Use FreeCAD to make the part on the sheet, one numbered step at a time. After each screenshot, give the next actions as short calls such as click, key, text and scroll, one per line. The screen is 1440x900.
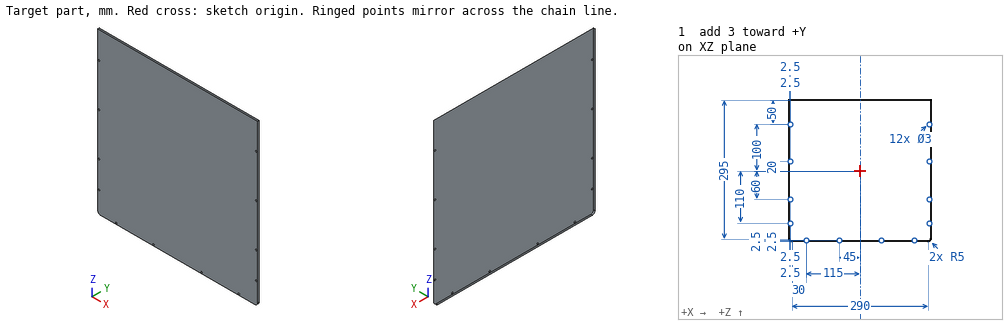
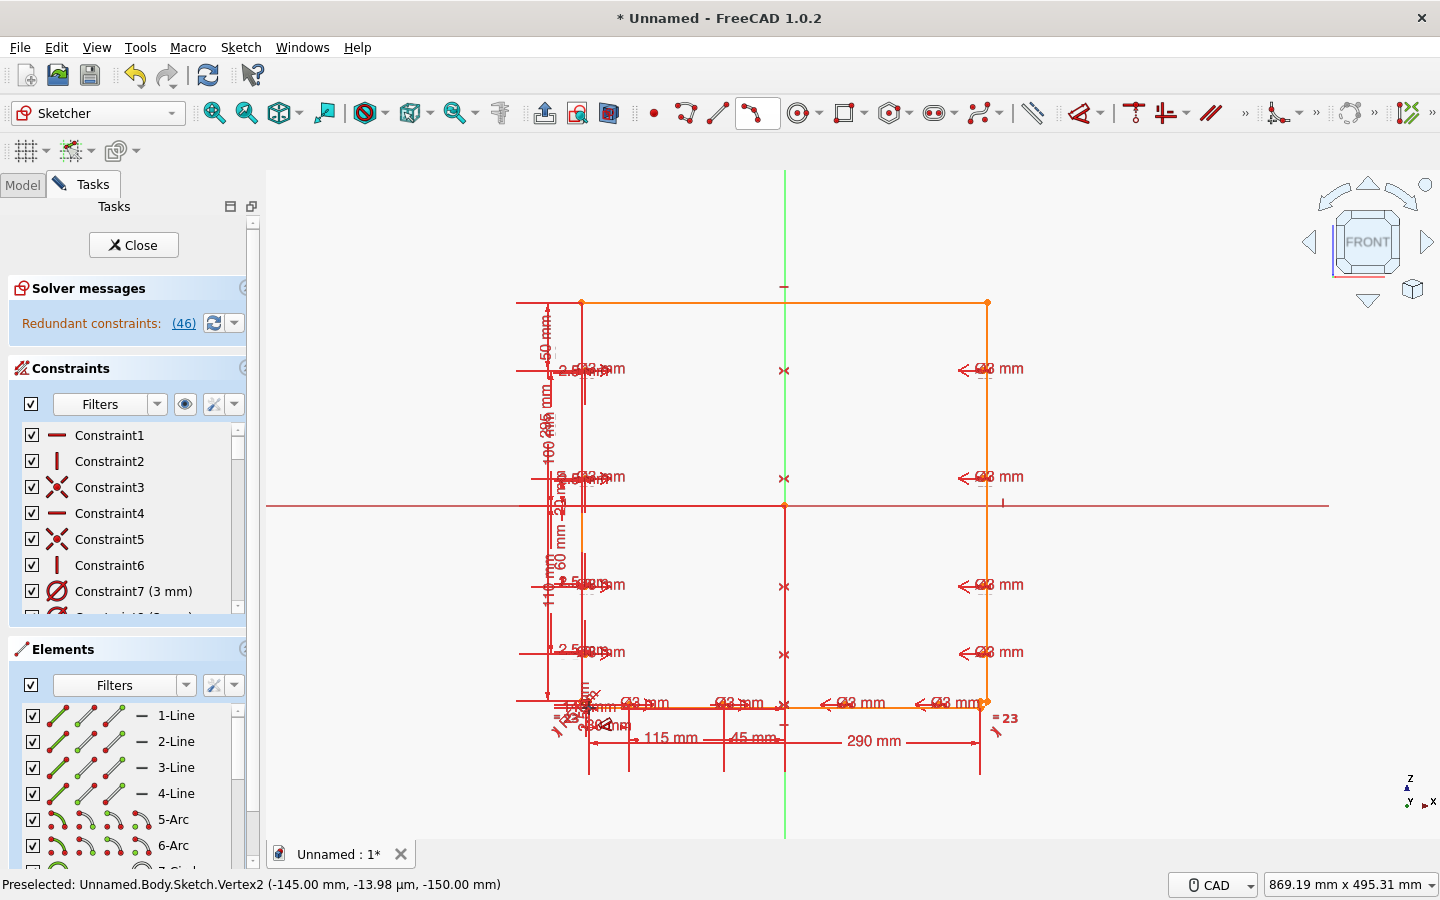
scroll(724, 705, up, 13)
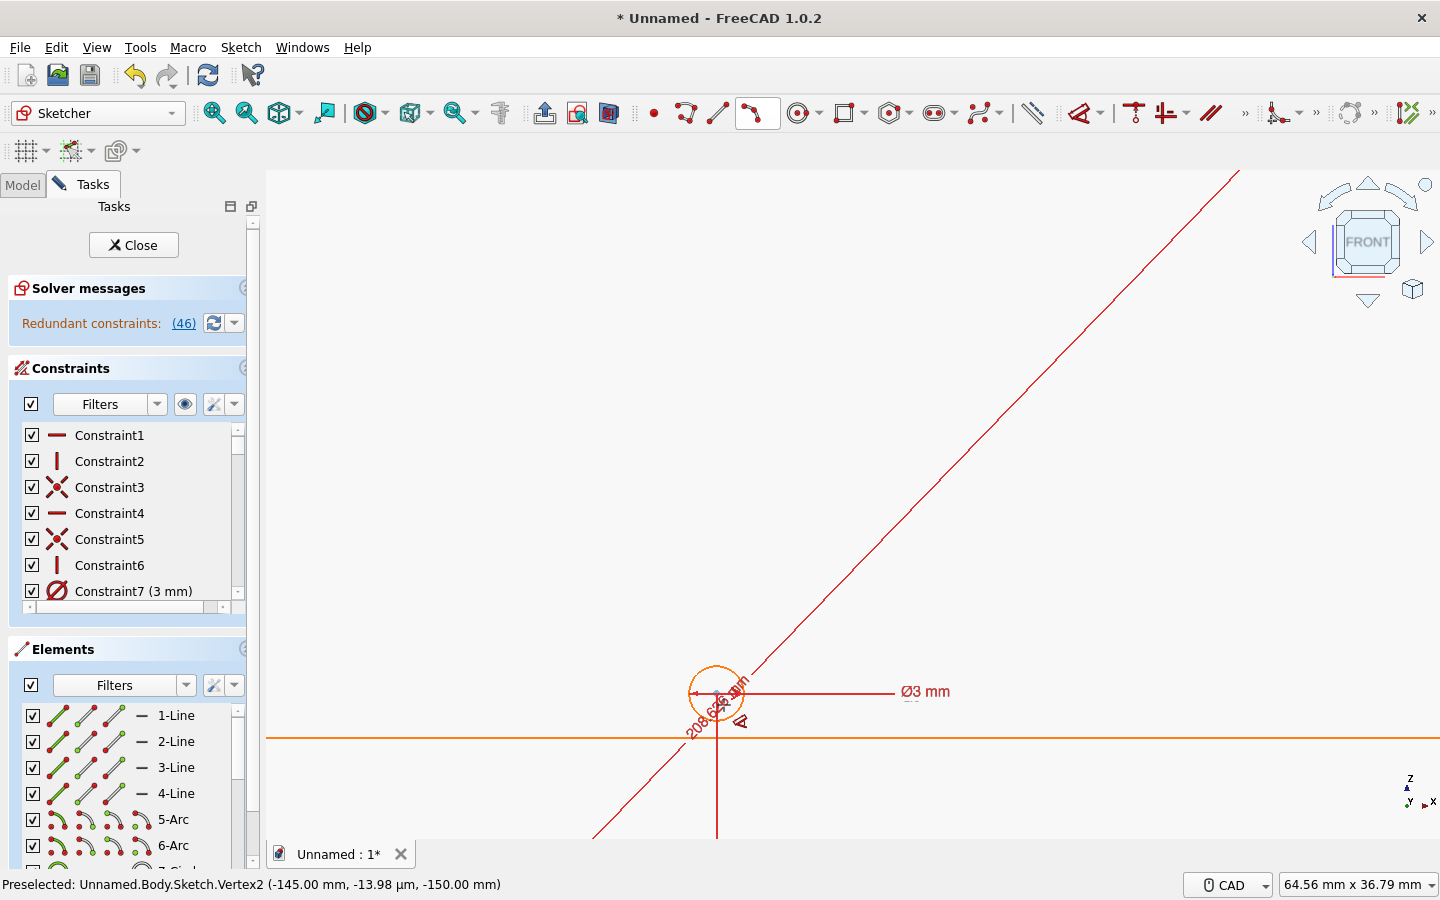
click(717, 694)
click(751, 716)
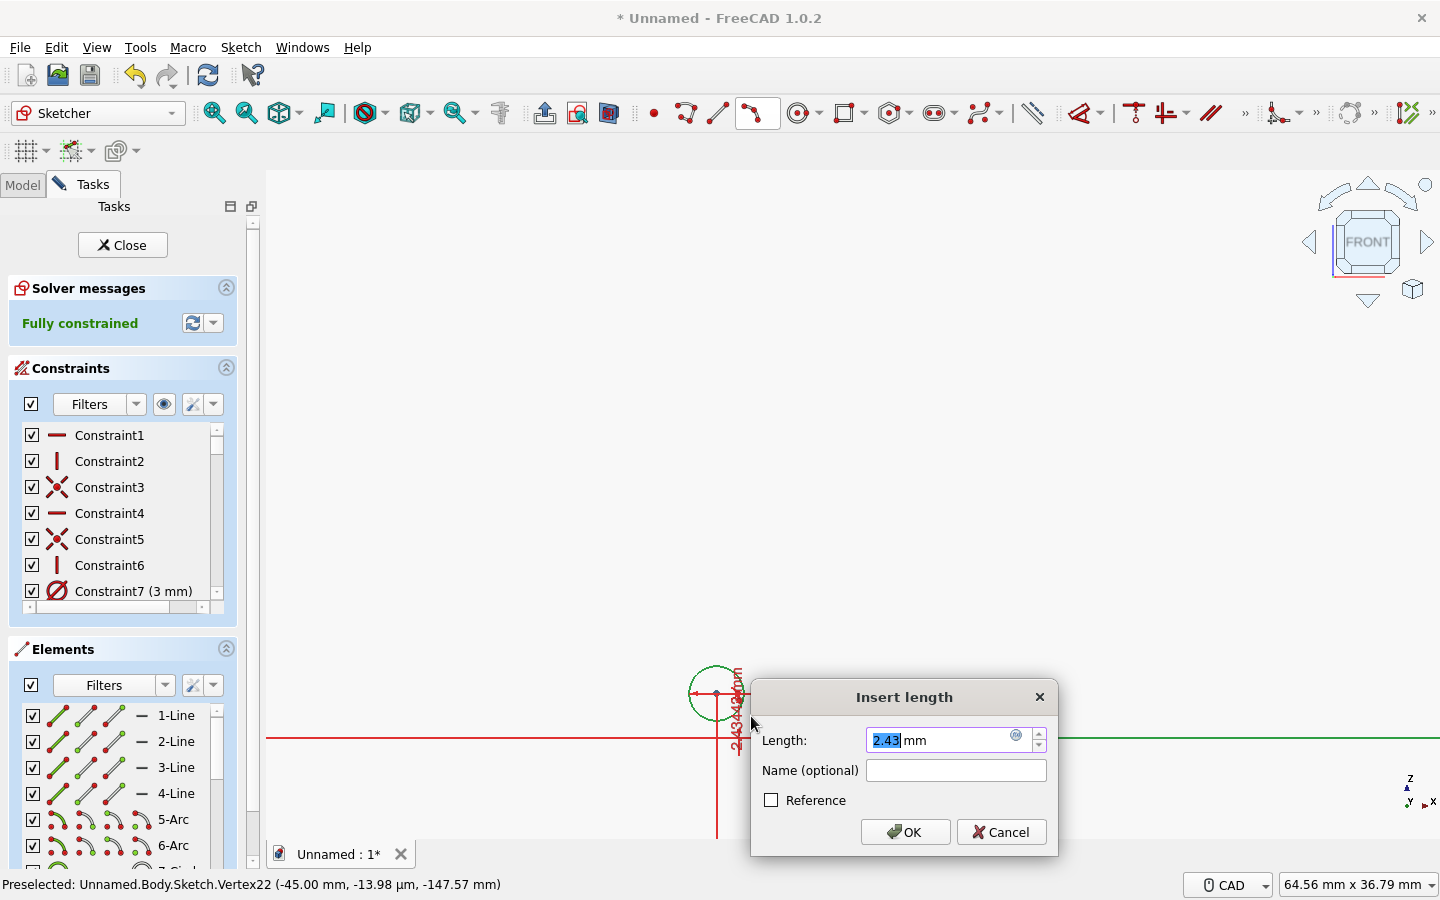
text(2.5)
key(Return)
key(Escape)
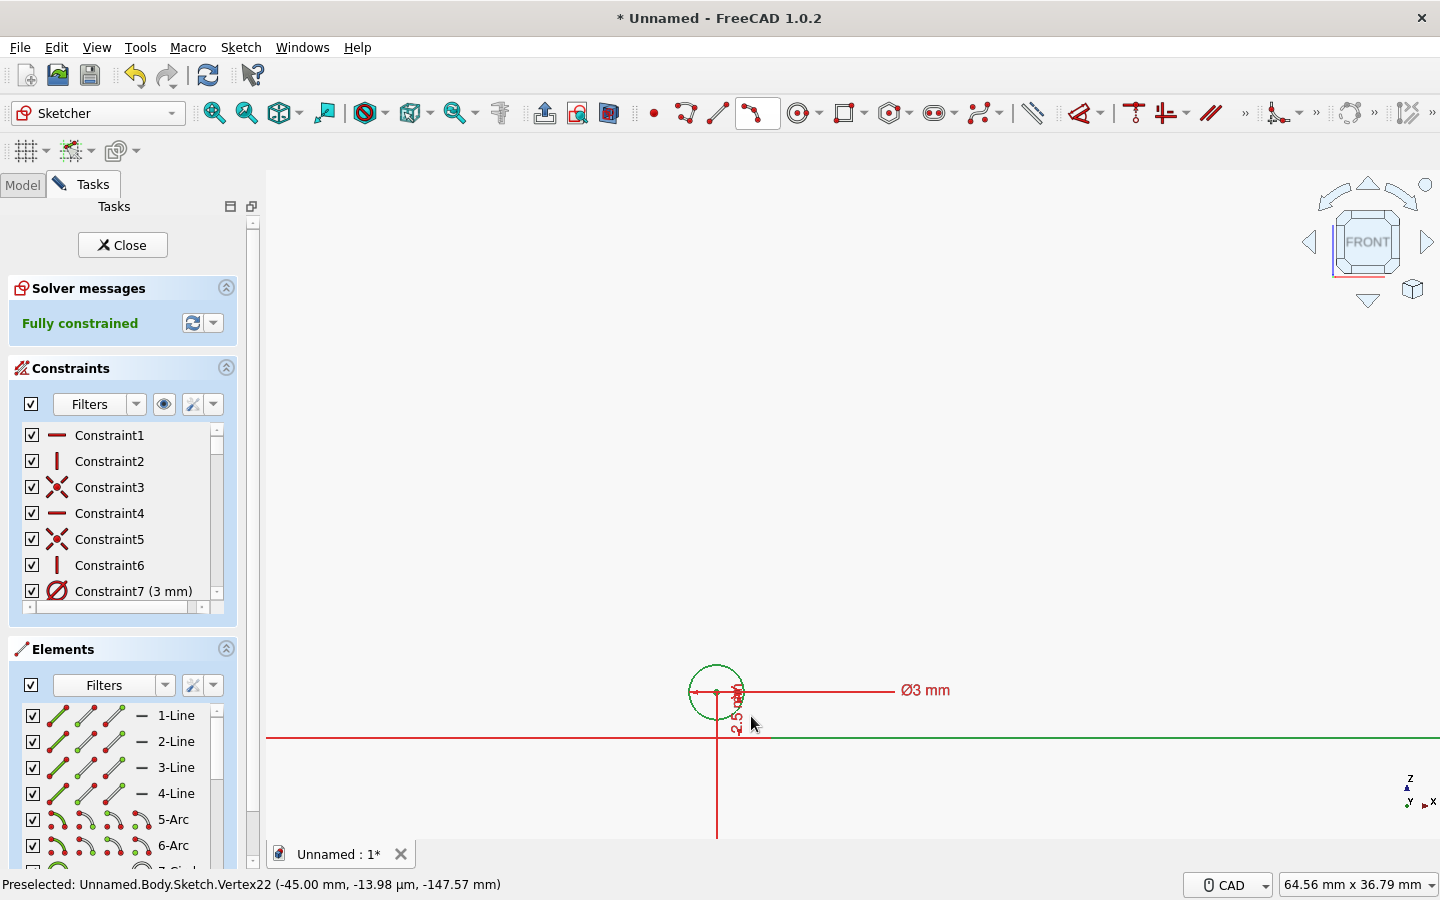
click(123, 245)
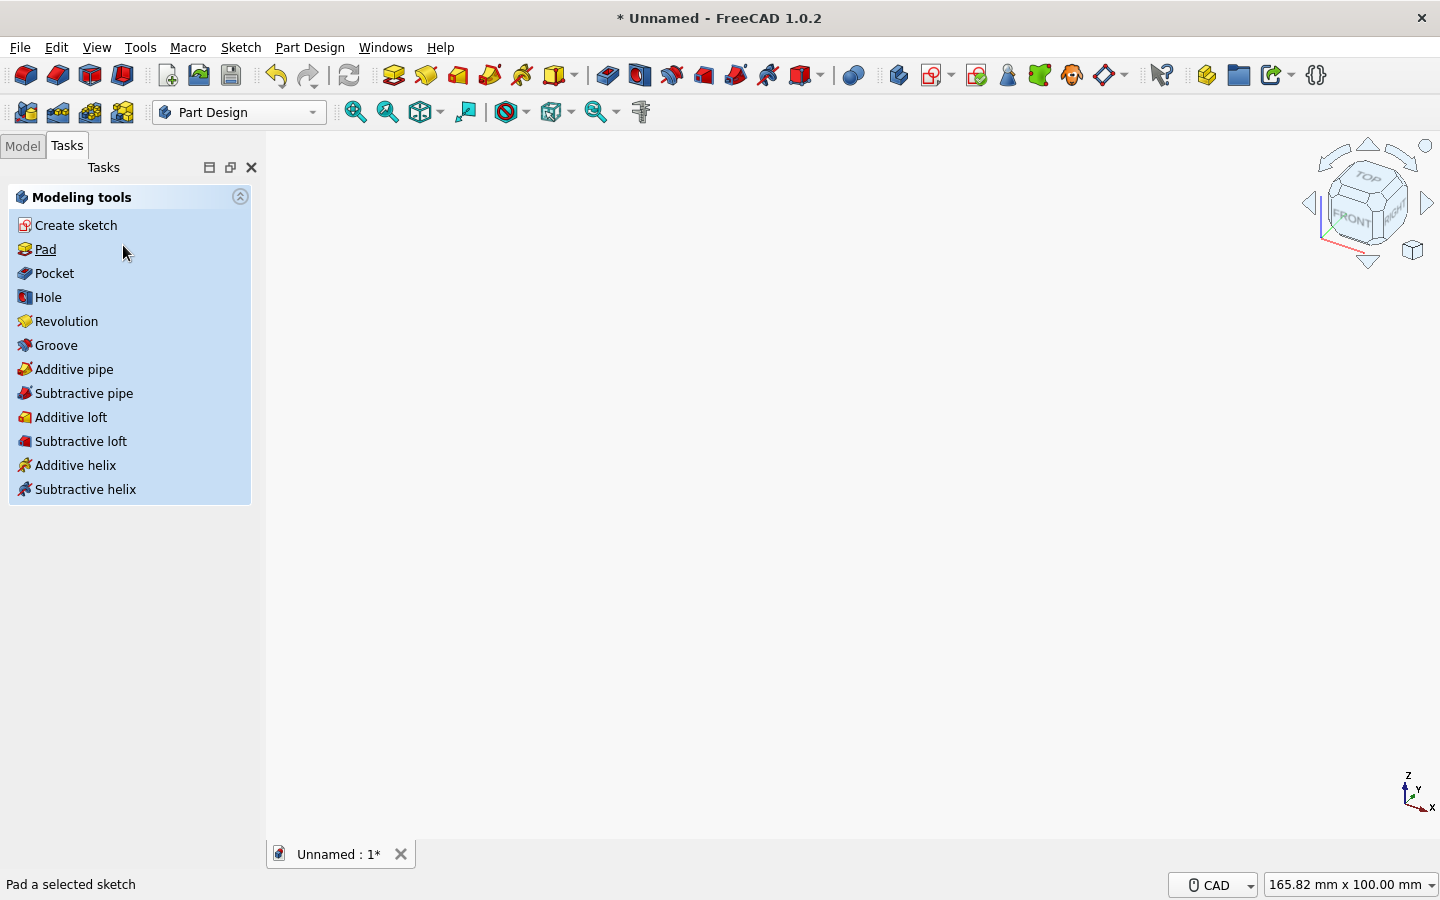
click(394, 76)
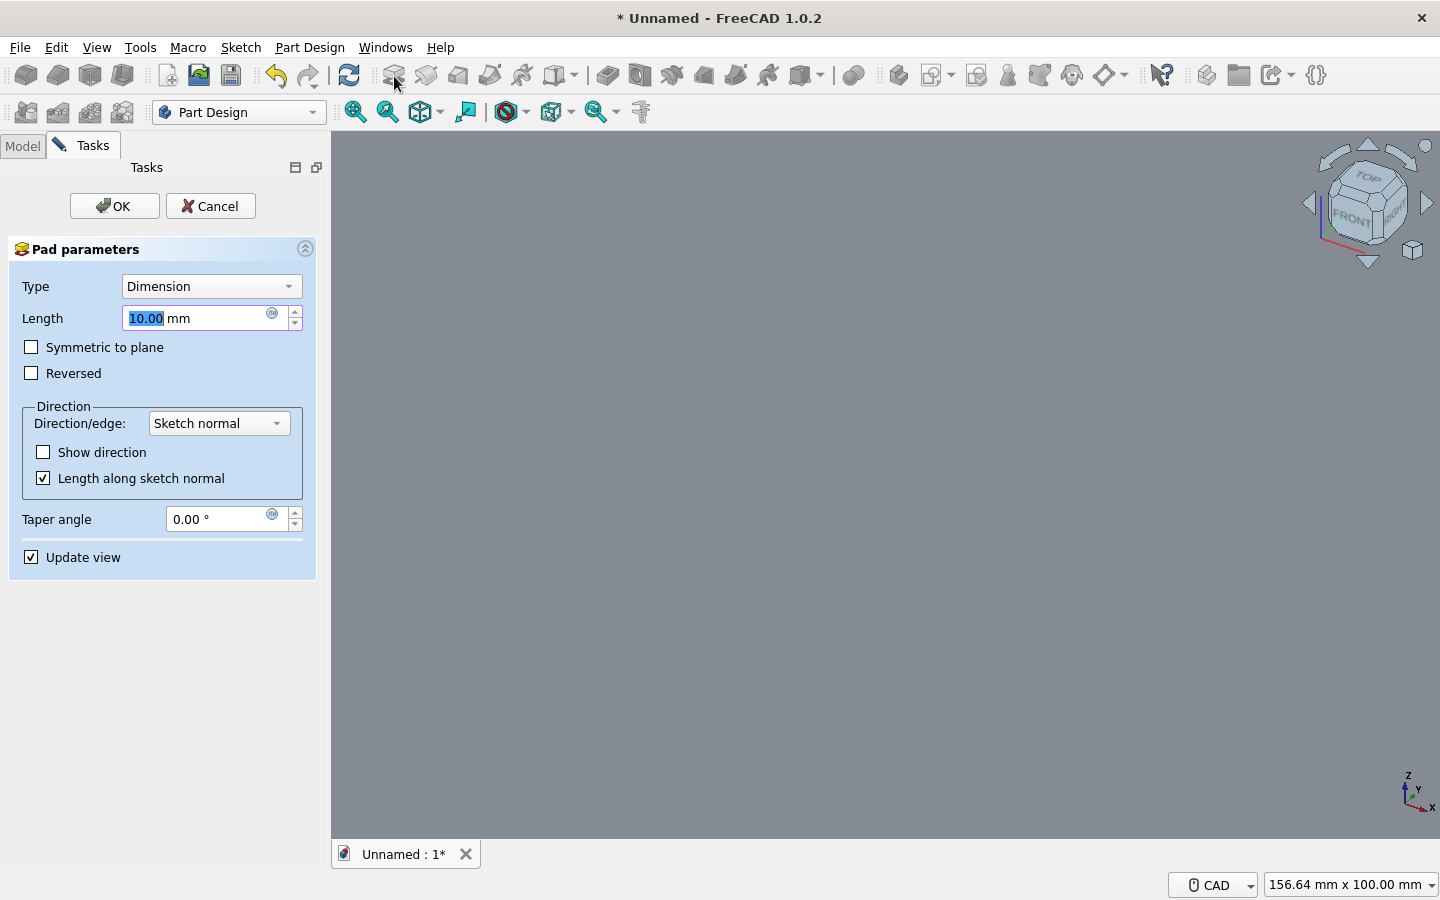
text(3)
key(Tab)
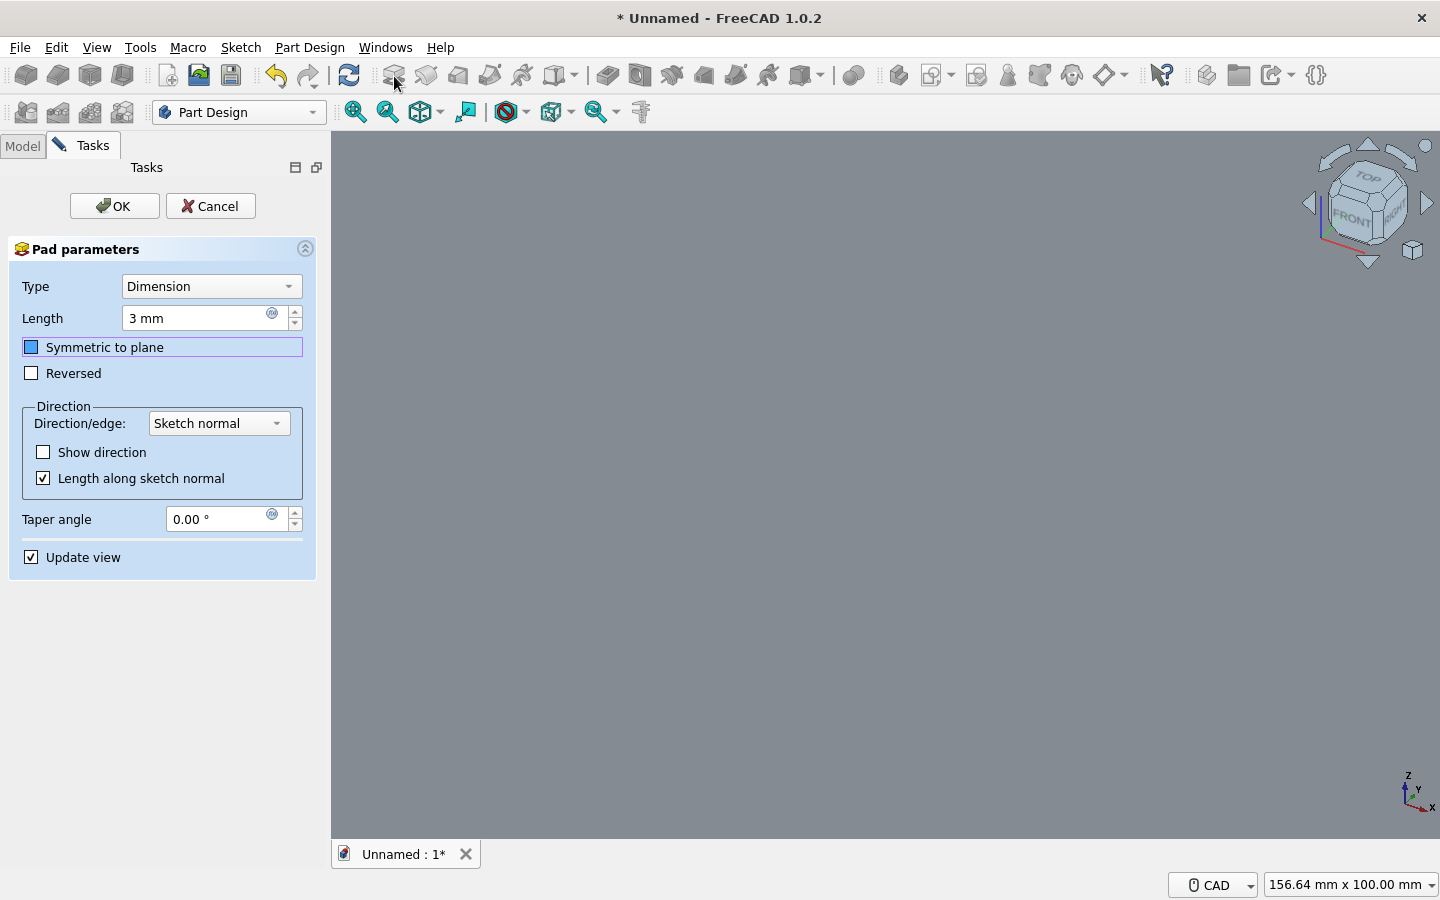
click(30, 373)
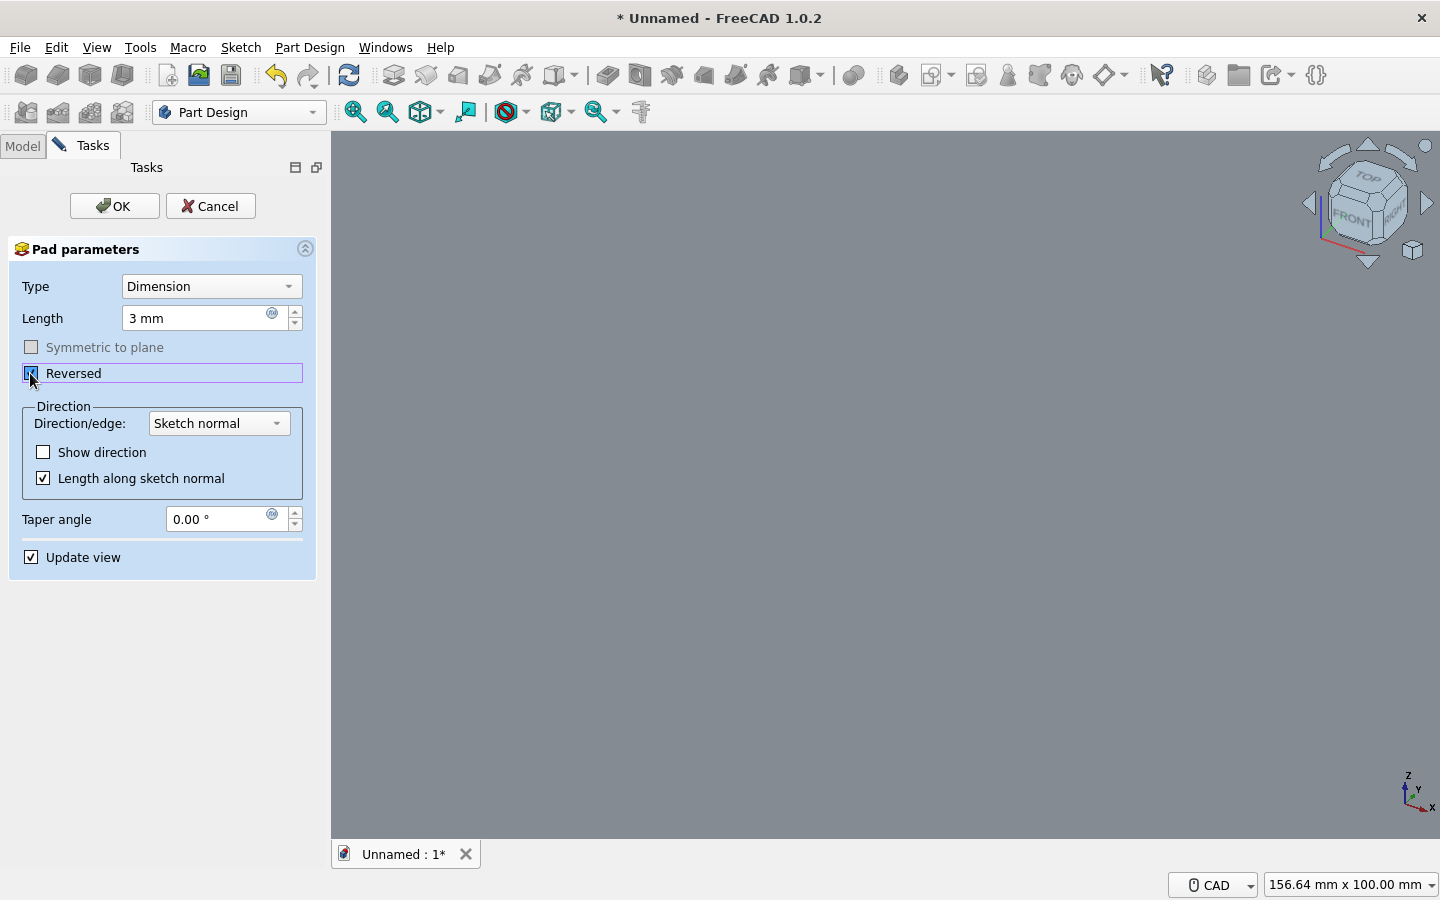
click(115, 206)